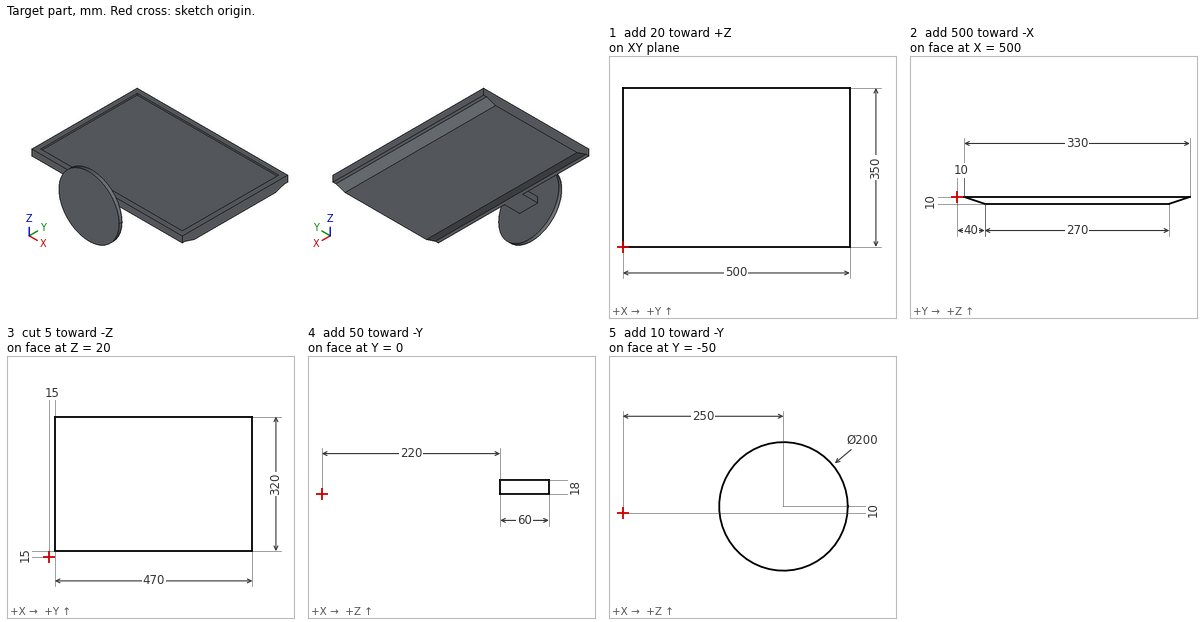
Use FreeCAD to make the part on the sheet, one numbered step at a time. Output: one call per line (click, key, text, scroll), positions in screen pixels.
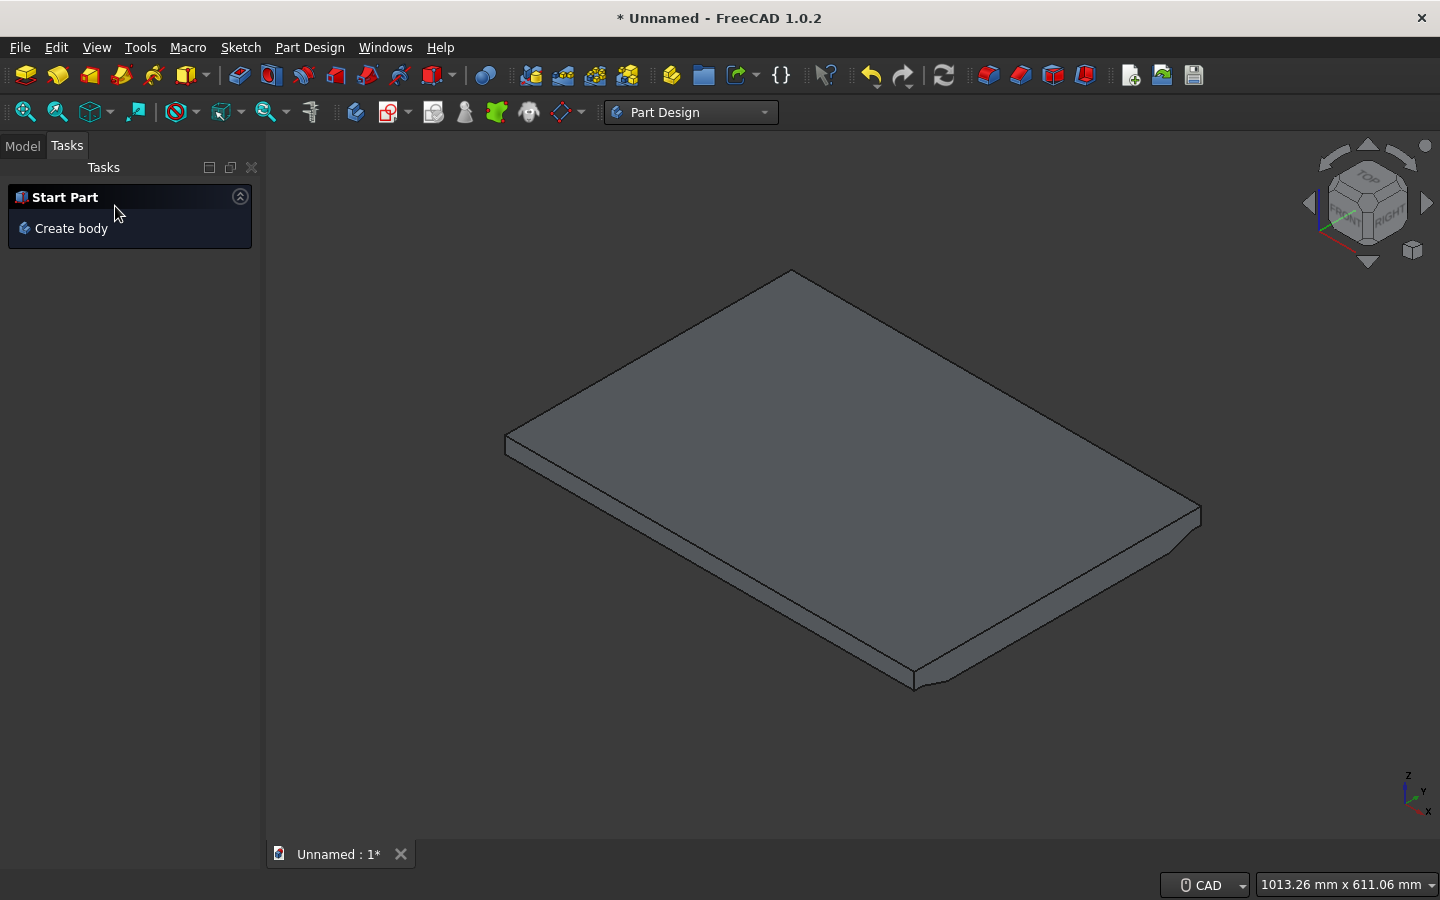
click(912, 504)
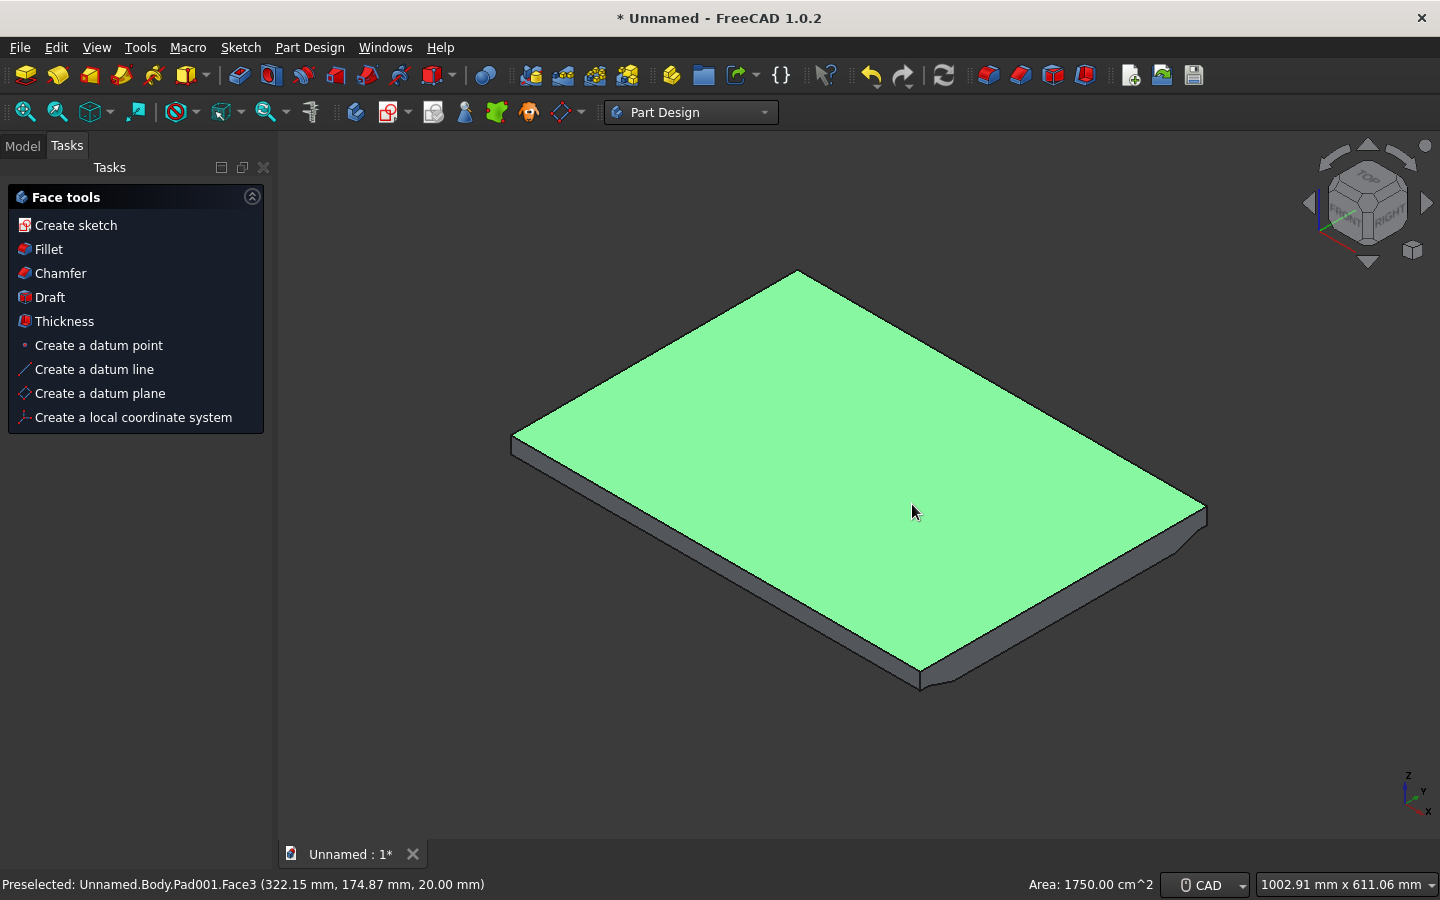
click(388, 112)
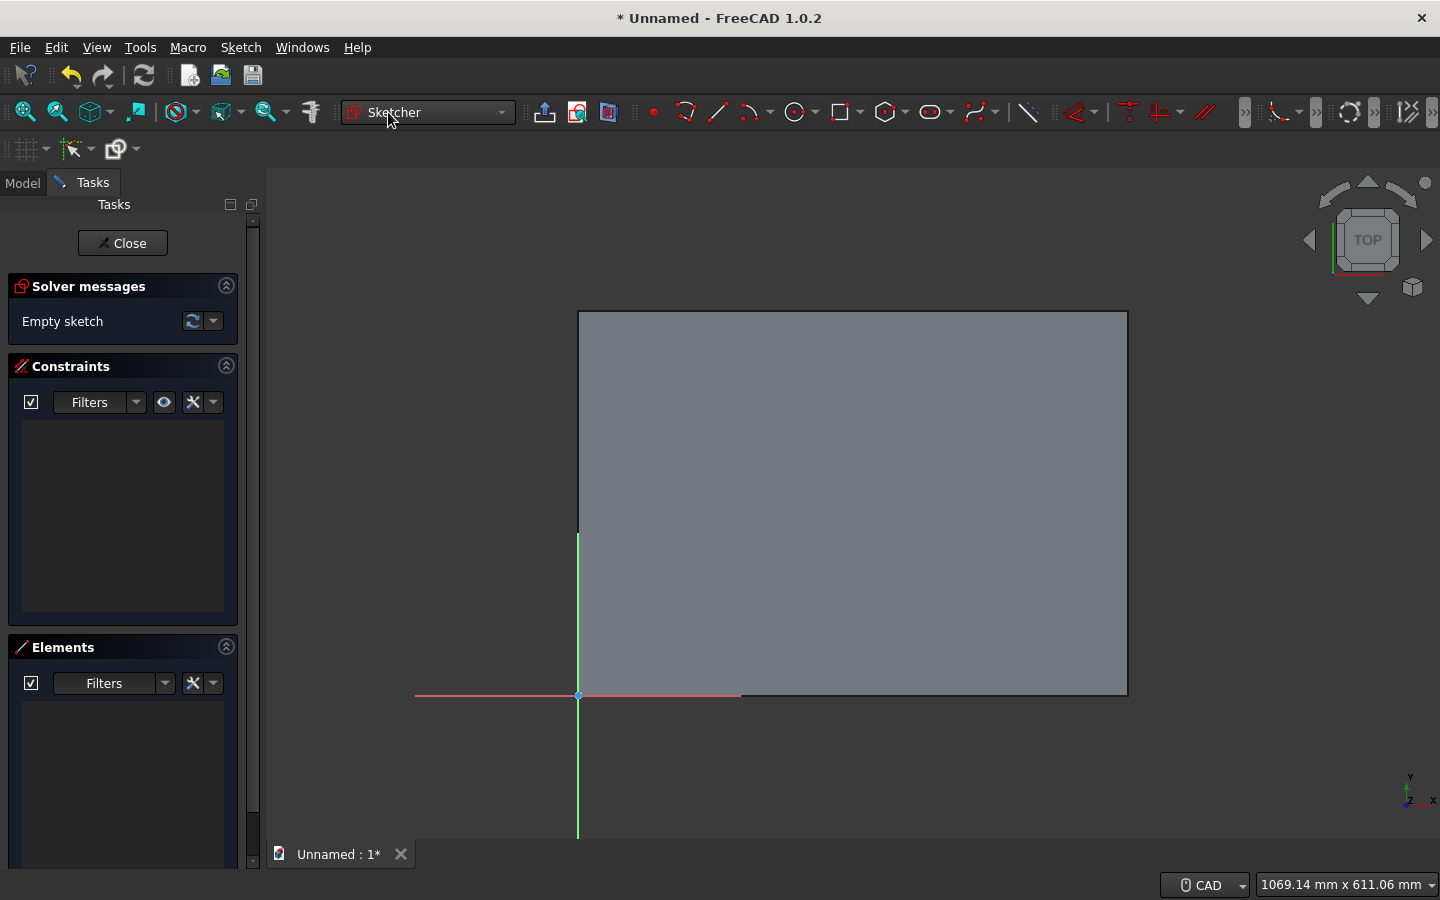
click(840, 112)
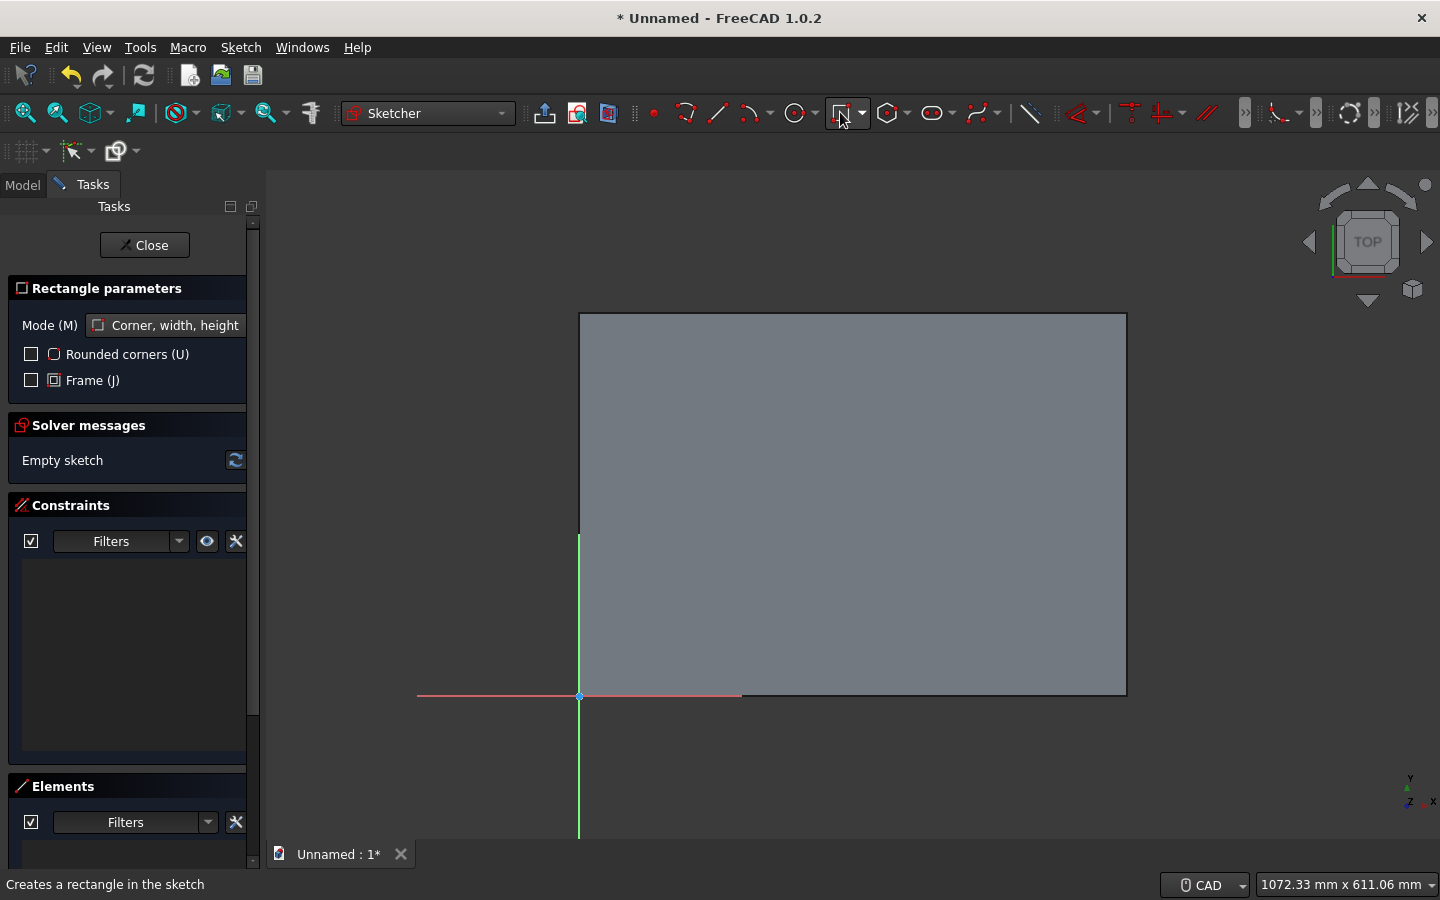
click(596, 329)
move(1110, 680)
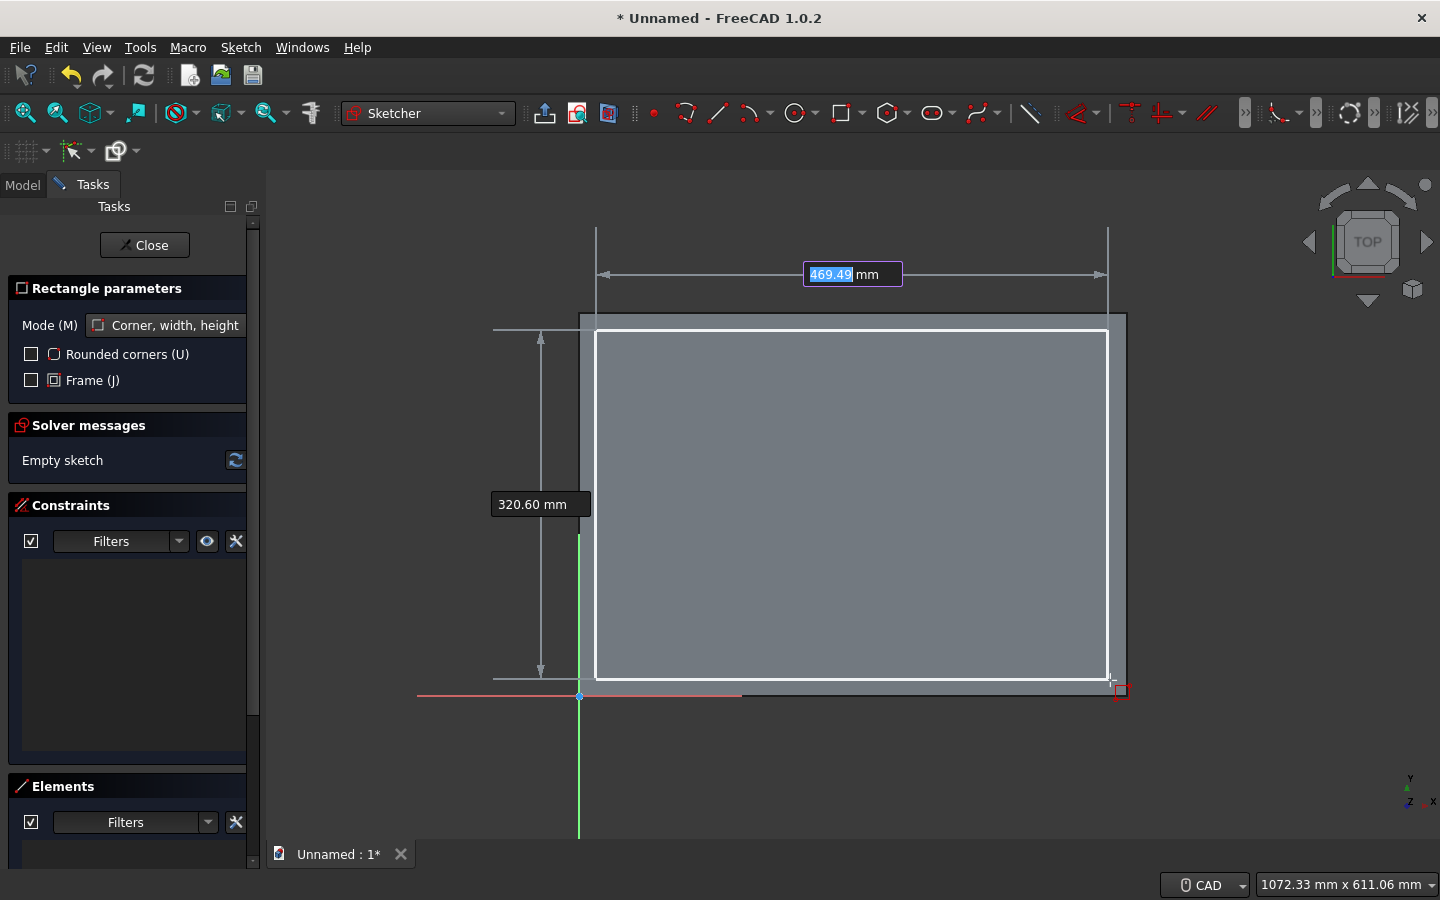
text(470)
key(Tab)
text(320)
key(Return)
key(Escape)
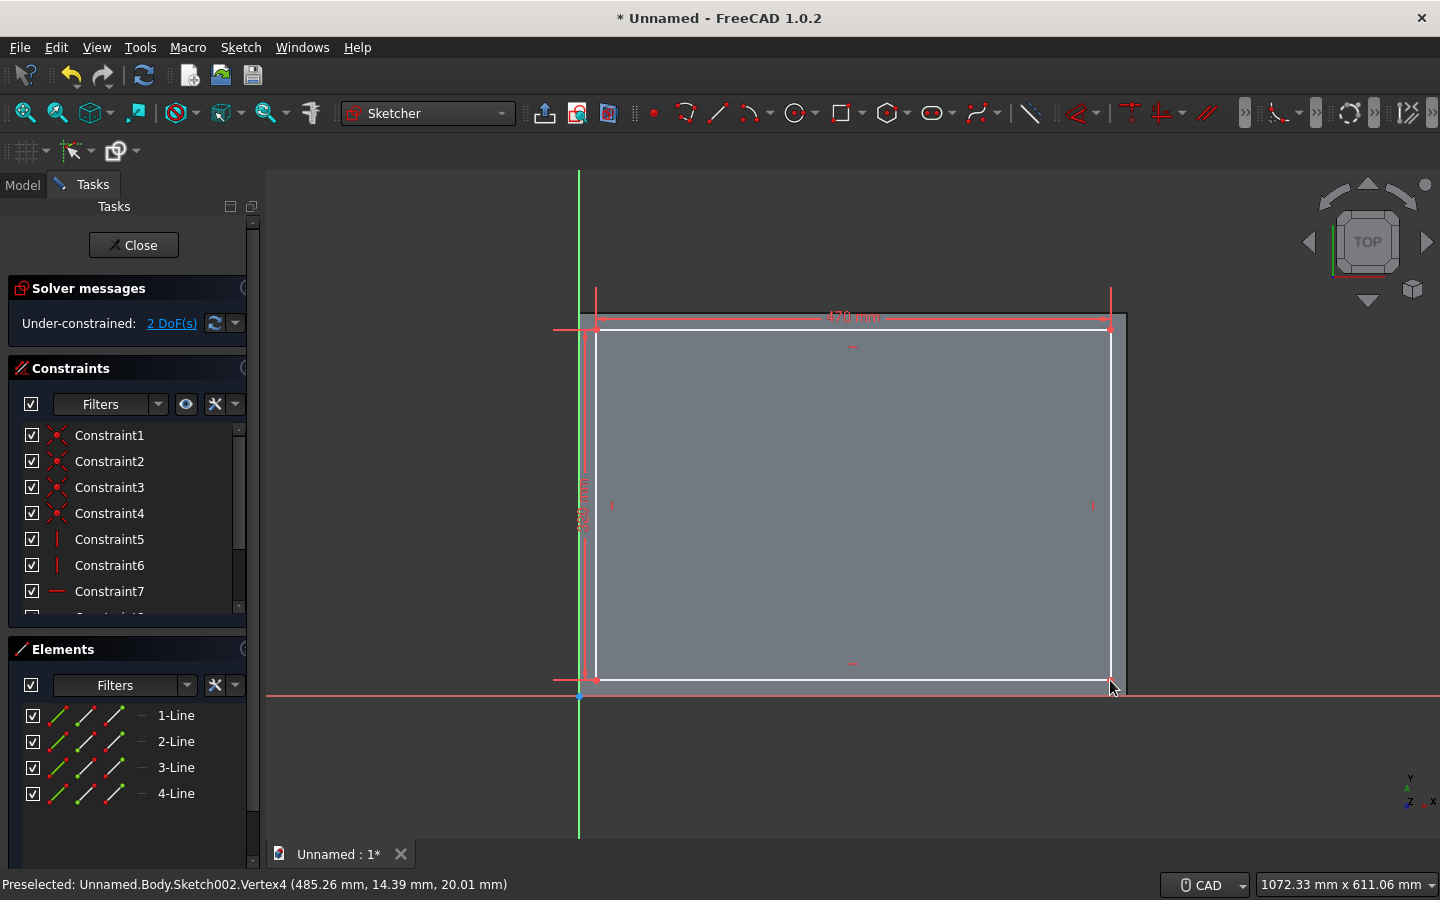
click(1076, 114)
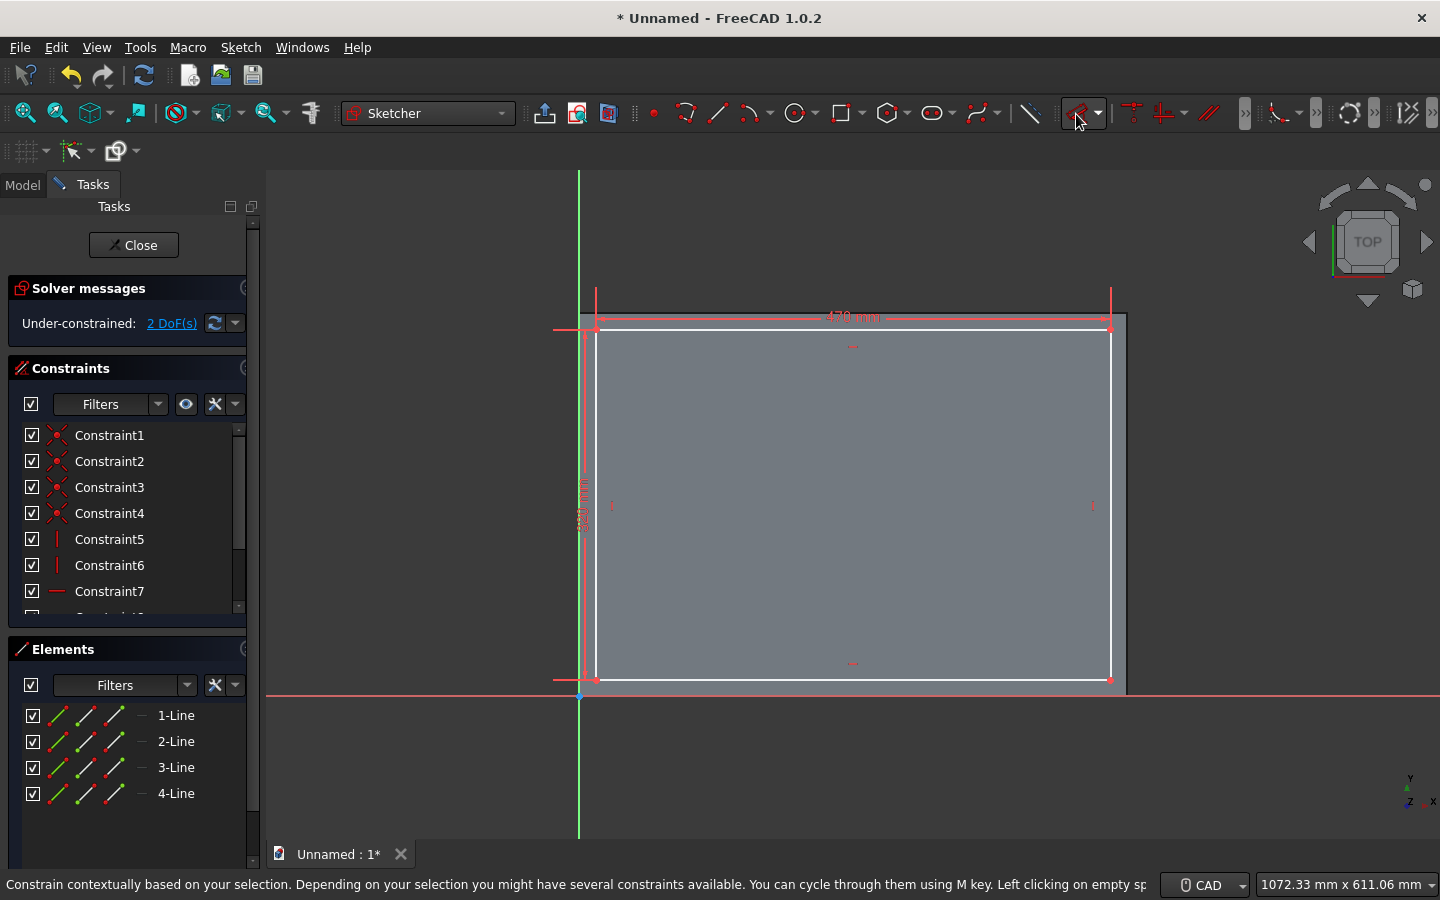
scroll(596, 330, up, 5)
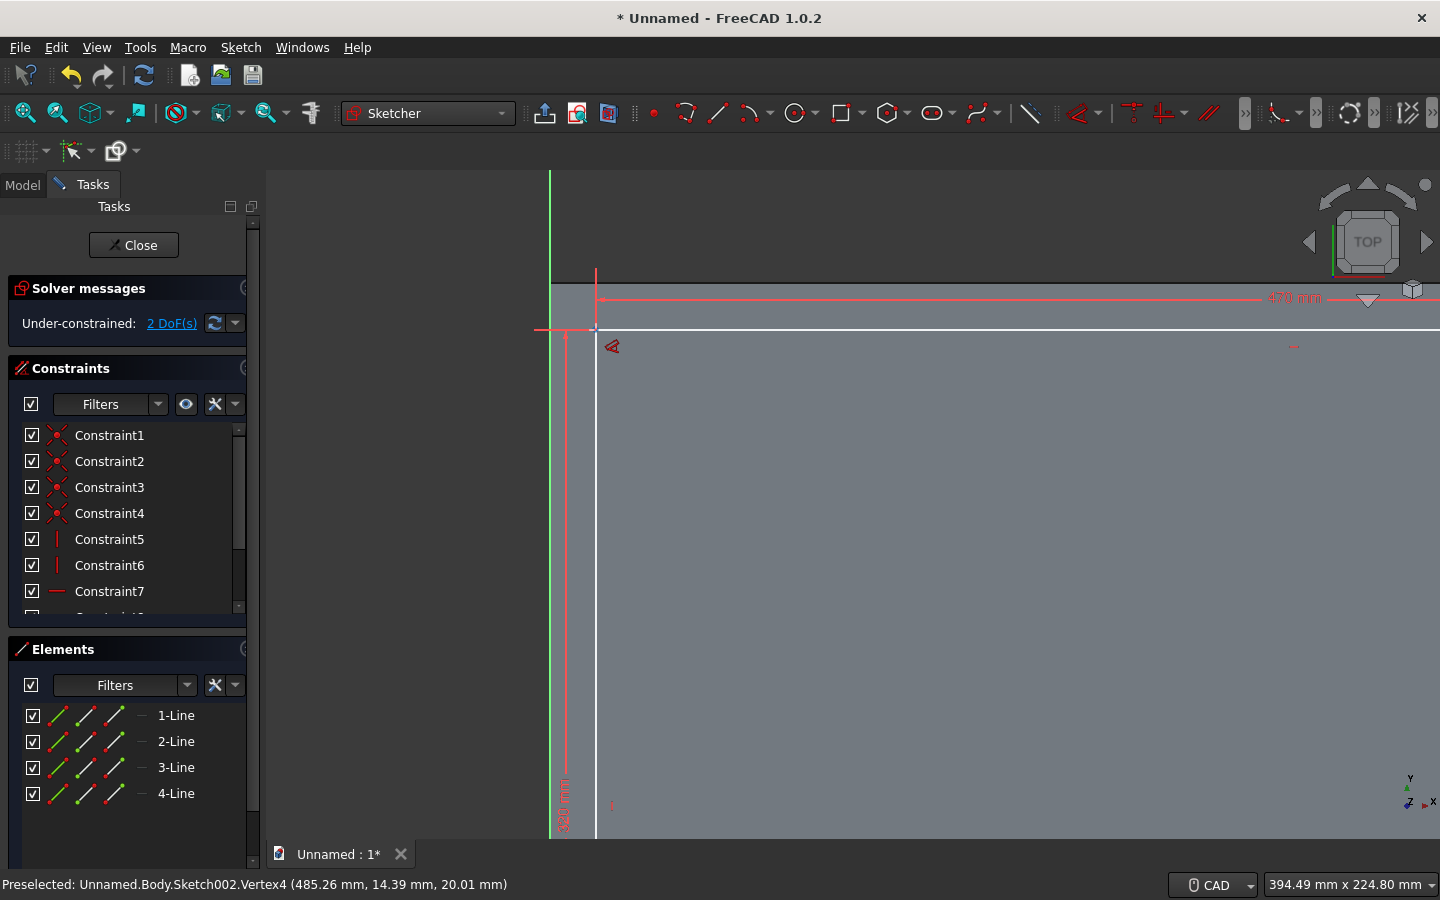
click(596, 330)
click(573, 296)